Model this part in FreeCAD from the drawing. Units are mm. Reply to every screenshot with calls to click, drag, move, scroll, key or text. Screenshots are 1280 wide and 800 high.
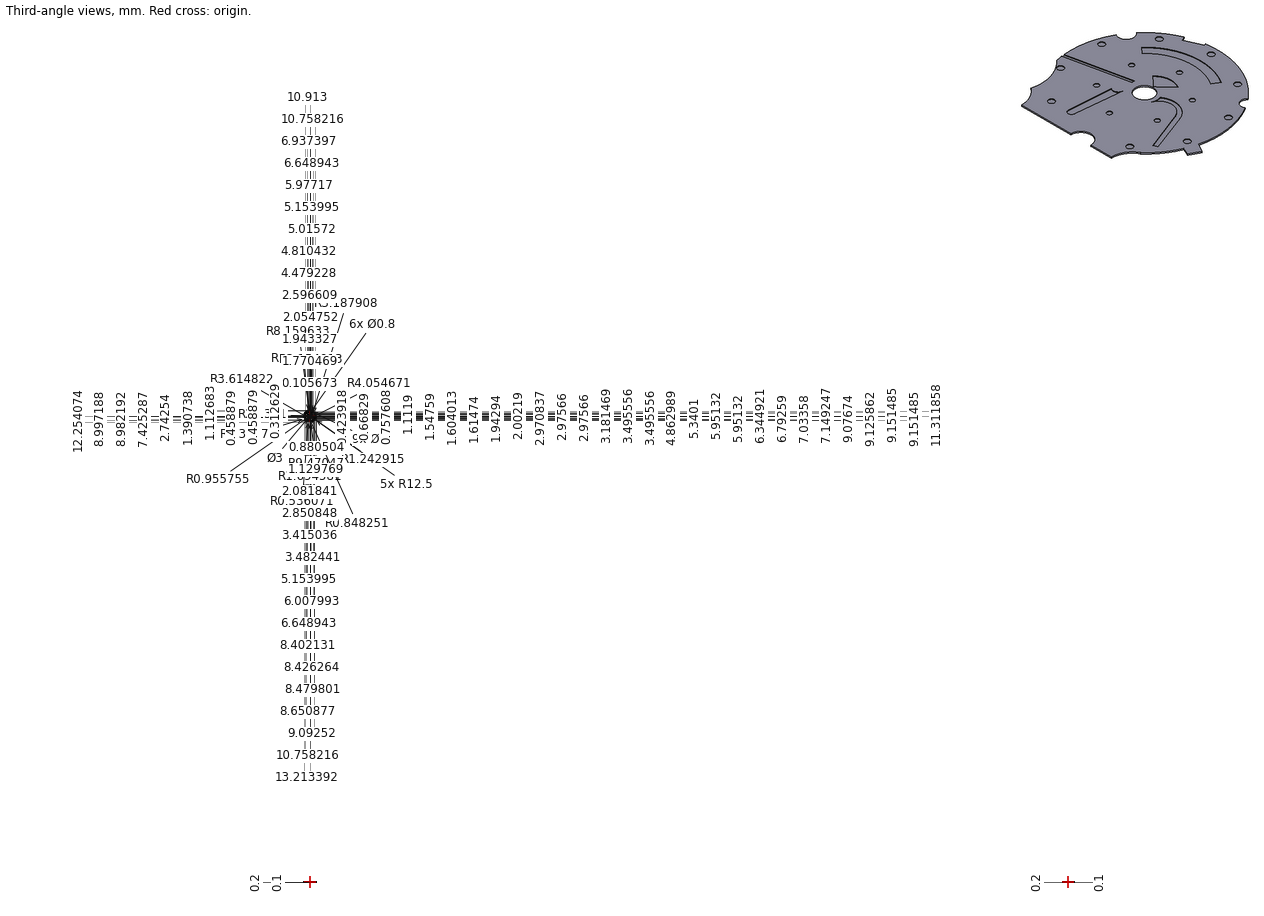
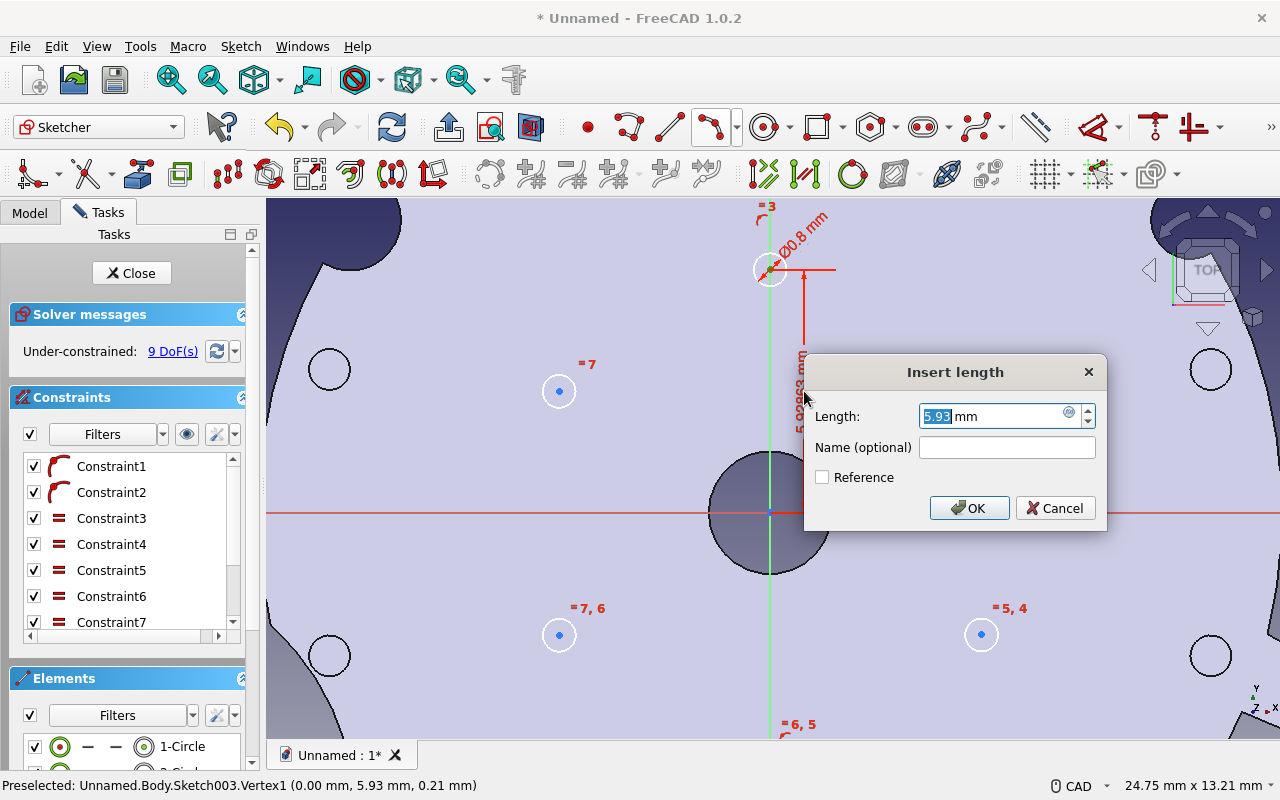
text(5.95132)
key(Return)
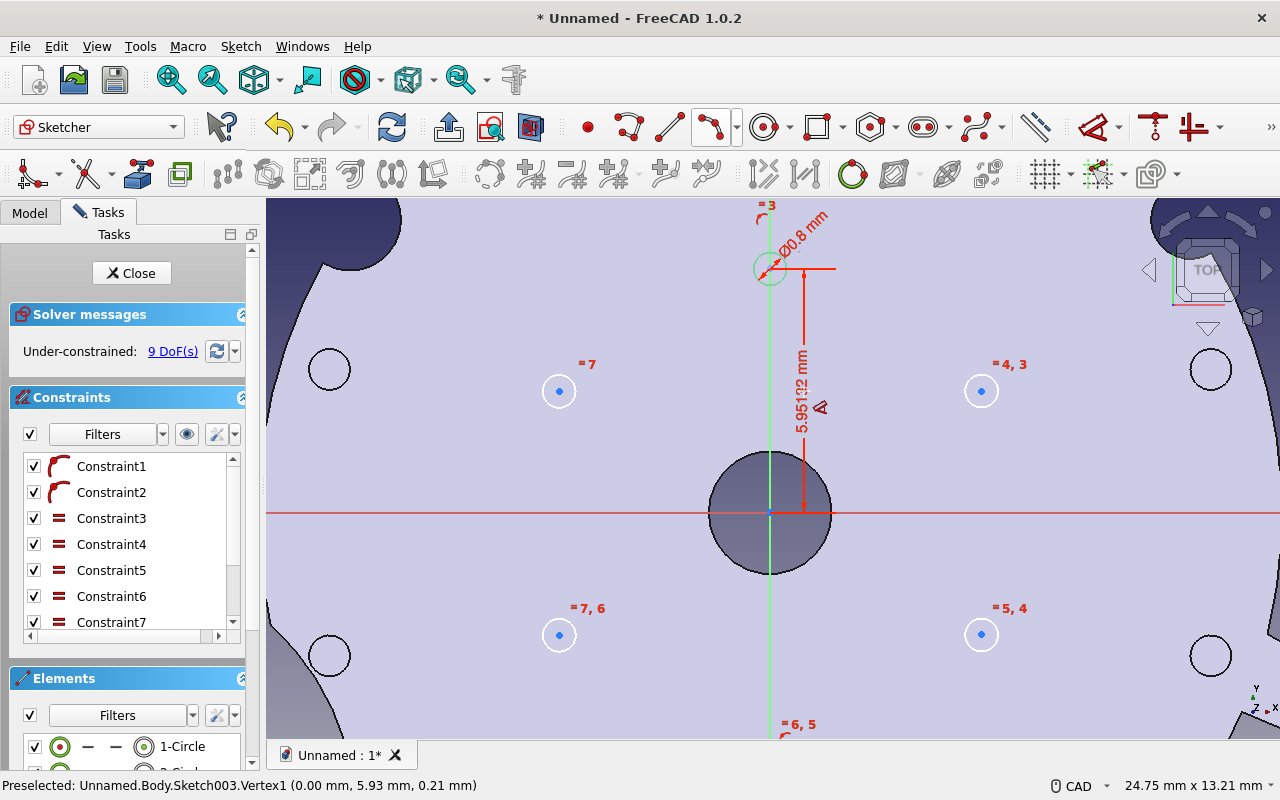
click(982, 391)
click(1016, 452)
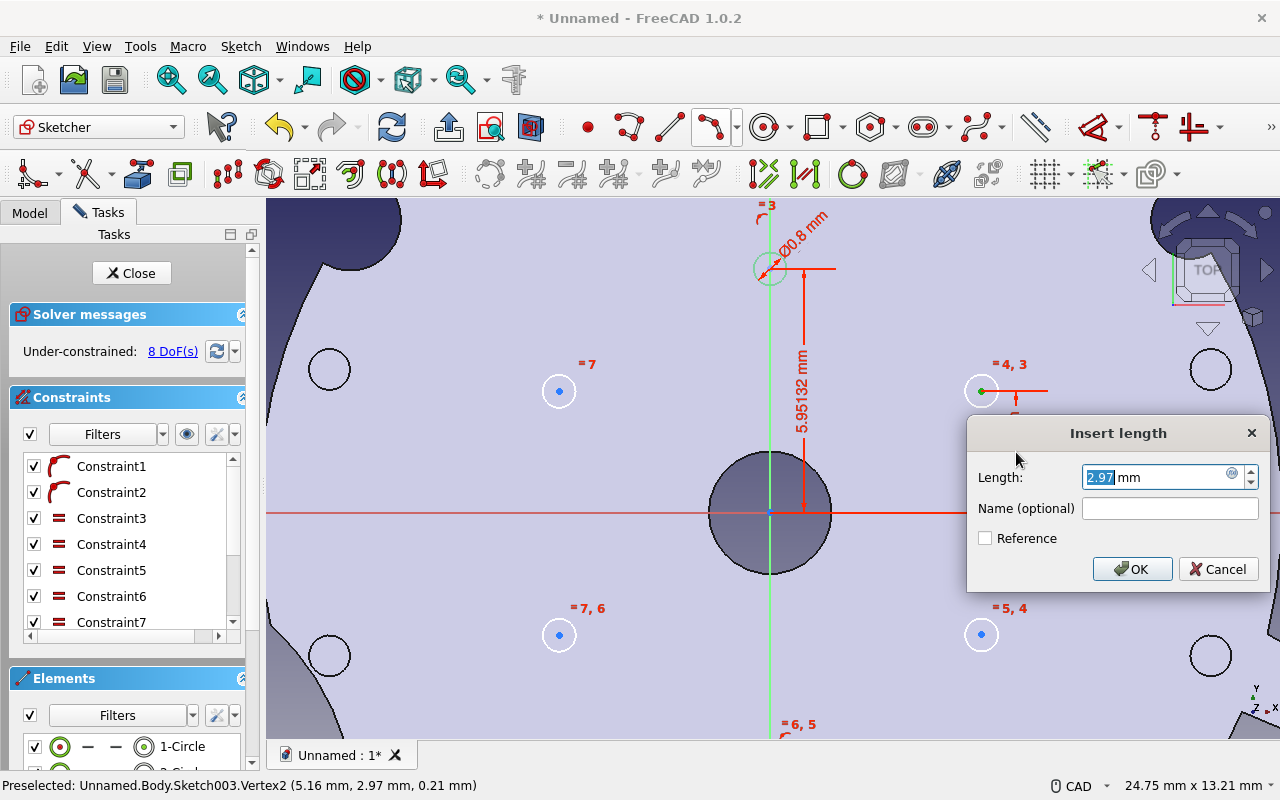
text(2.97566)
key(Return)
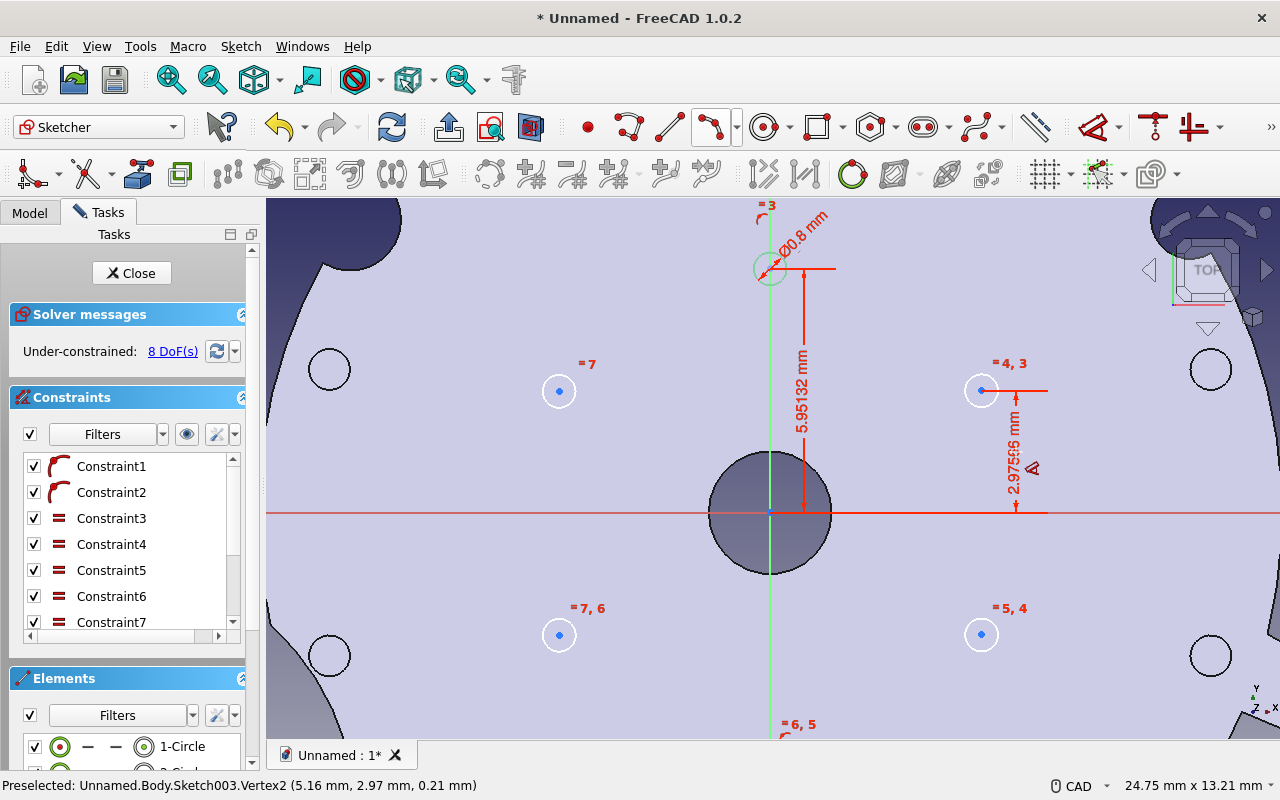
click(982, 635)
click(1016, 574)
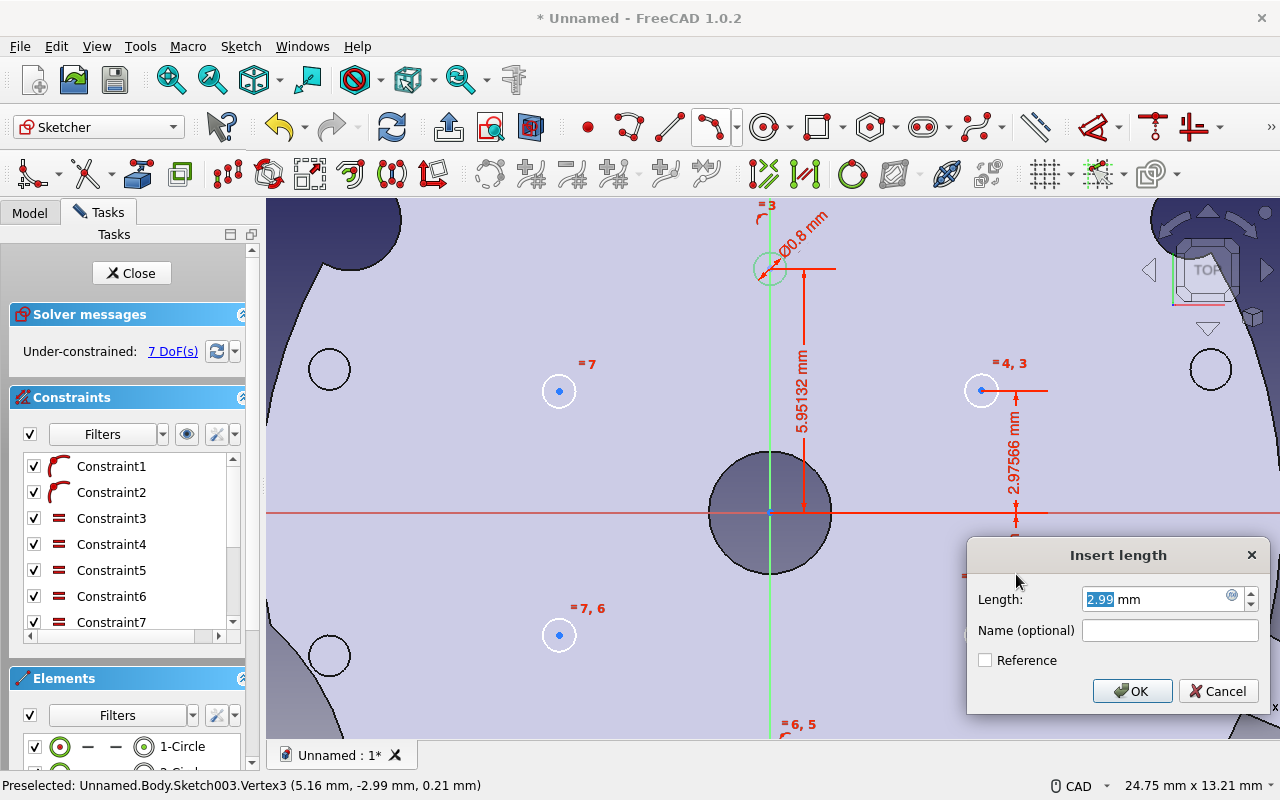
text(2.97566)
key(Return)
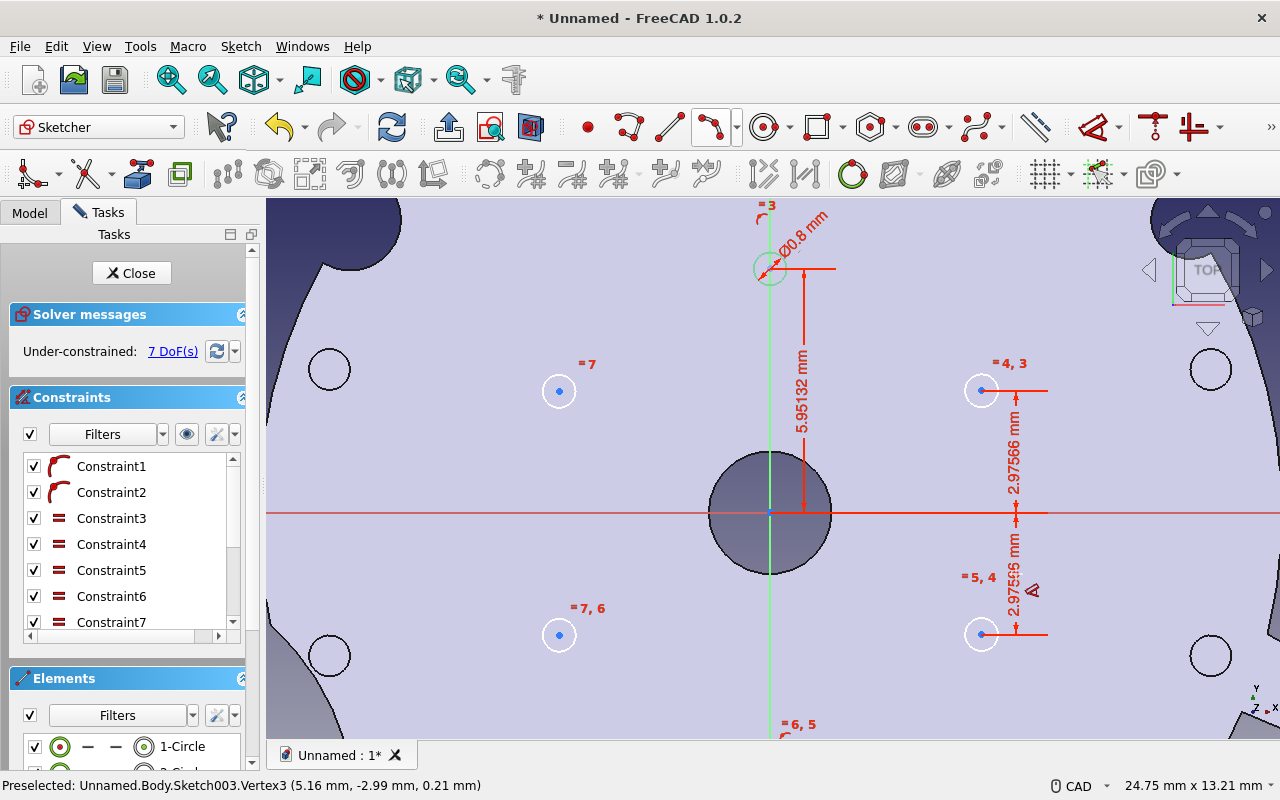
scroll(571, 379, down, 2)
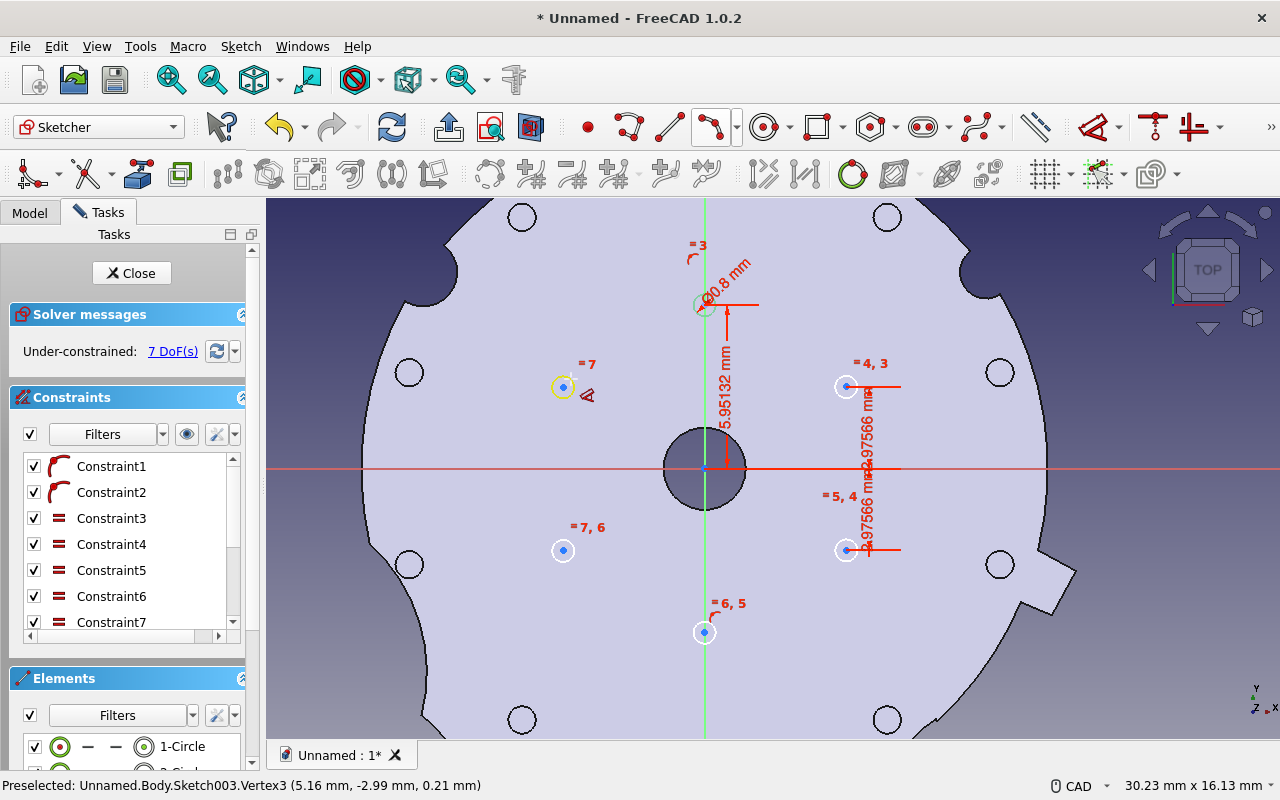
click(705, 633)
click(739, 551)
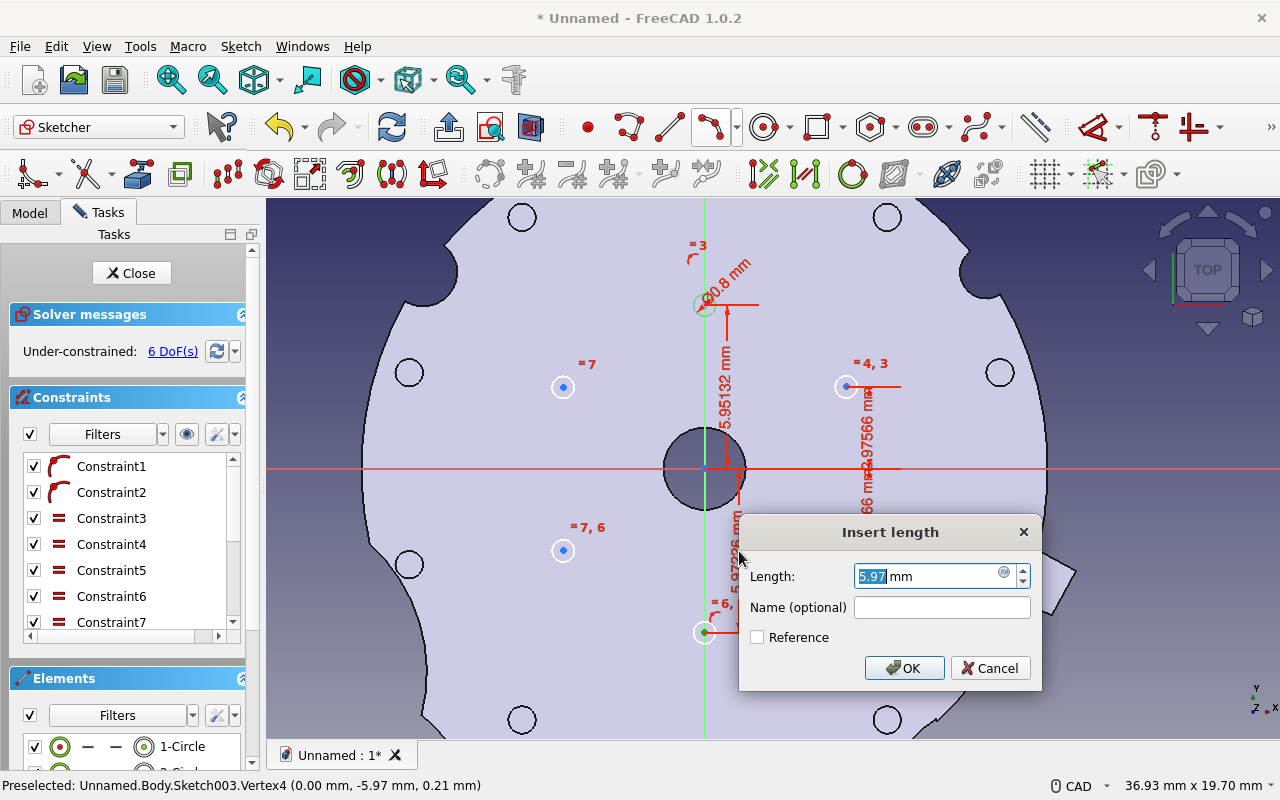
text(5.95132)
key(Return)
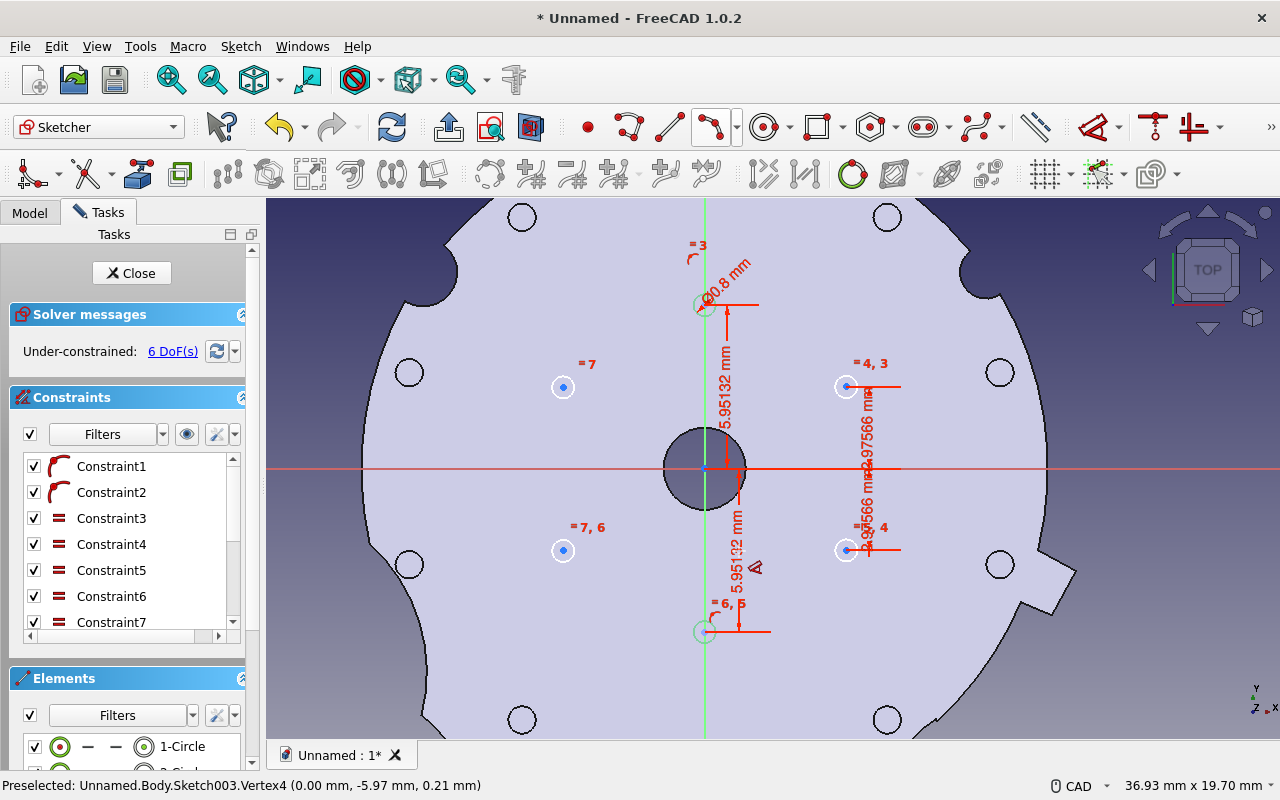
click(563, 551)
click(529, 510)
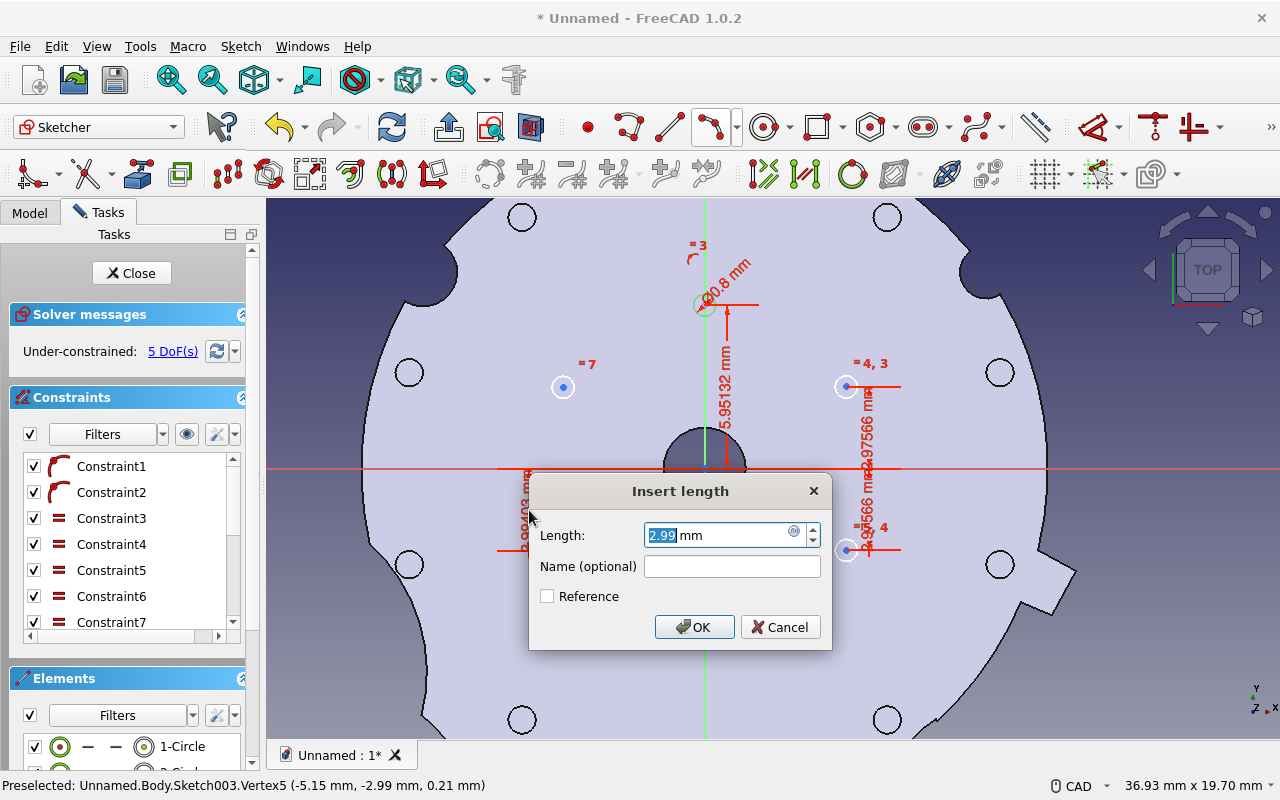
text(2.97566)
key(Return)